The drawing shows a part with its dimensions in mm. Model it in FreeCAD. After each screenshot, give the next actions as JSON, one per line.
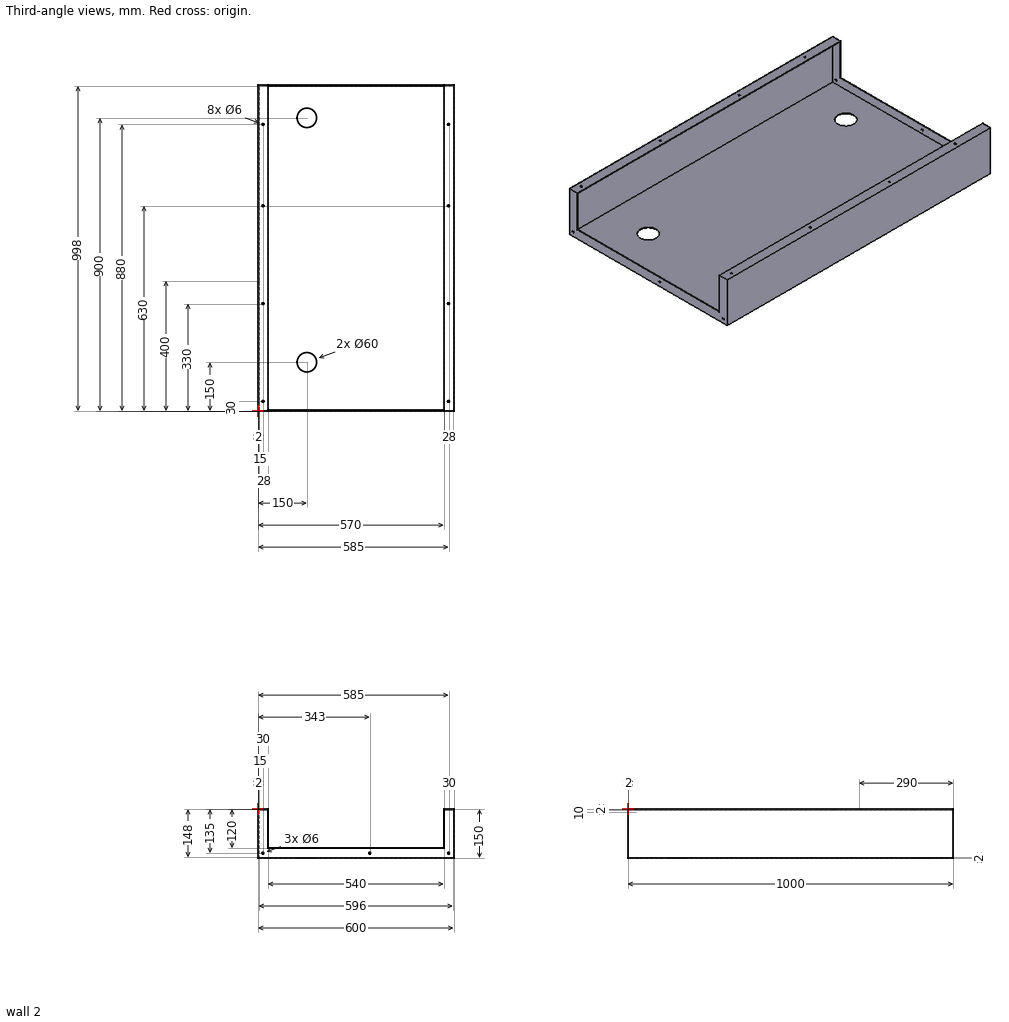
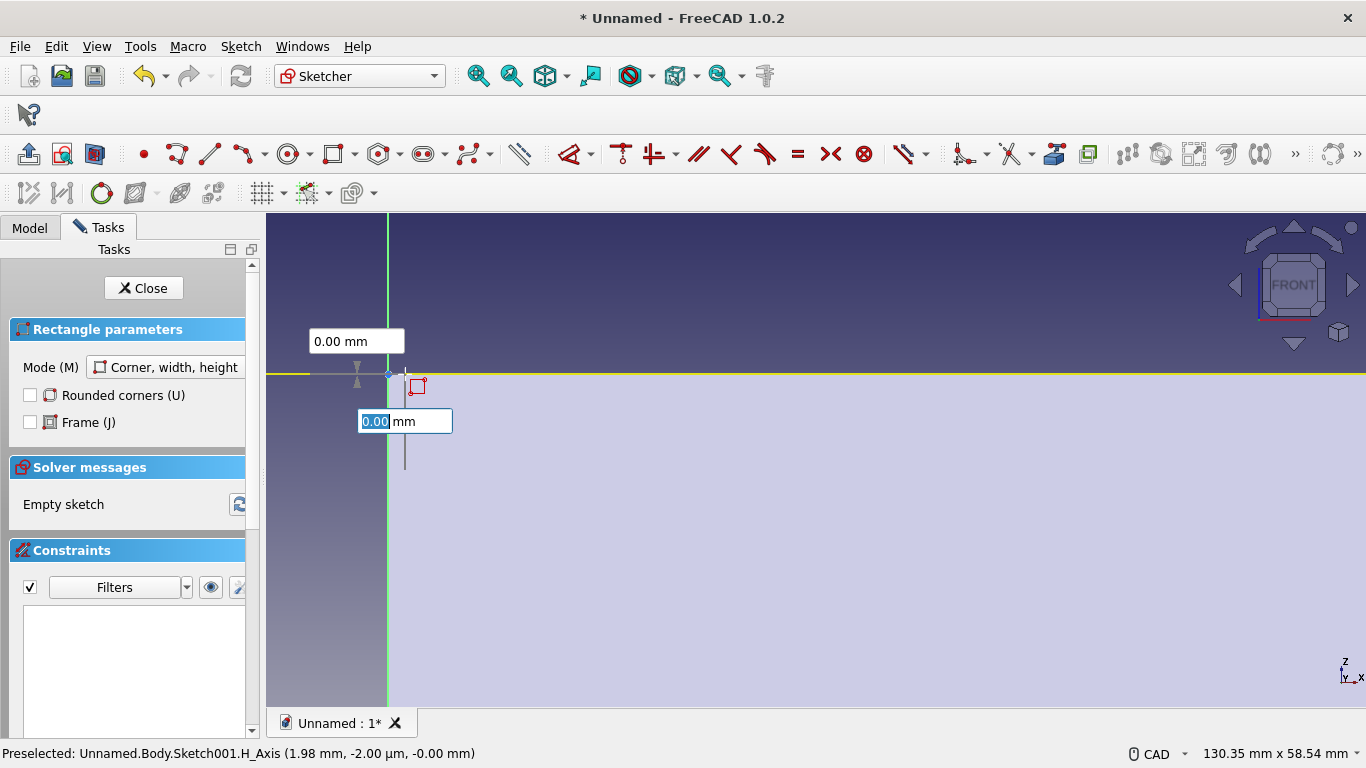
{"action": "scroll", "coordinate": [409, 376], "scroll_direction": "down", "scroll_amount": 10}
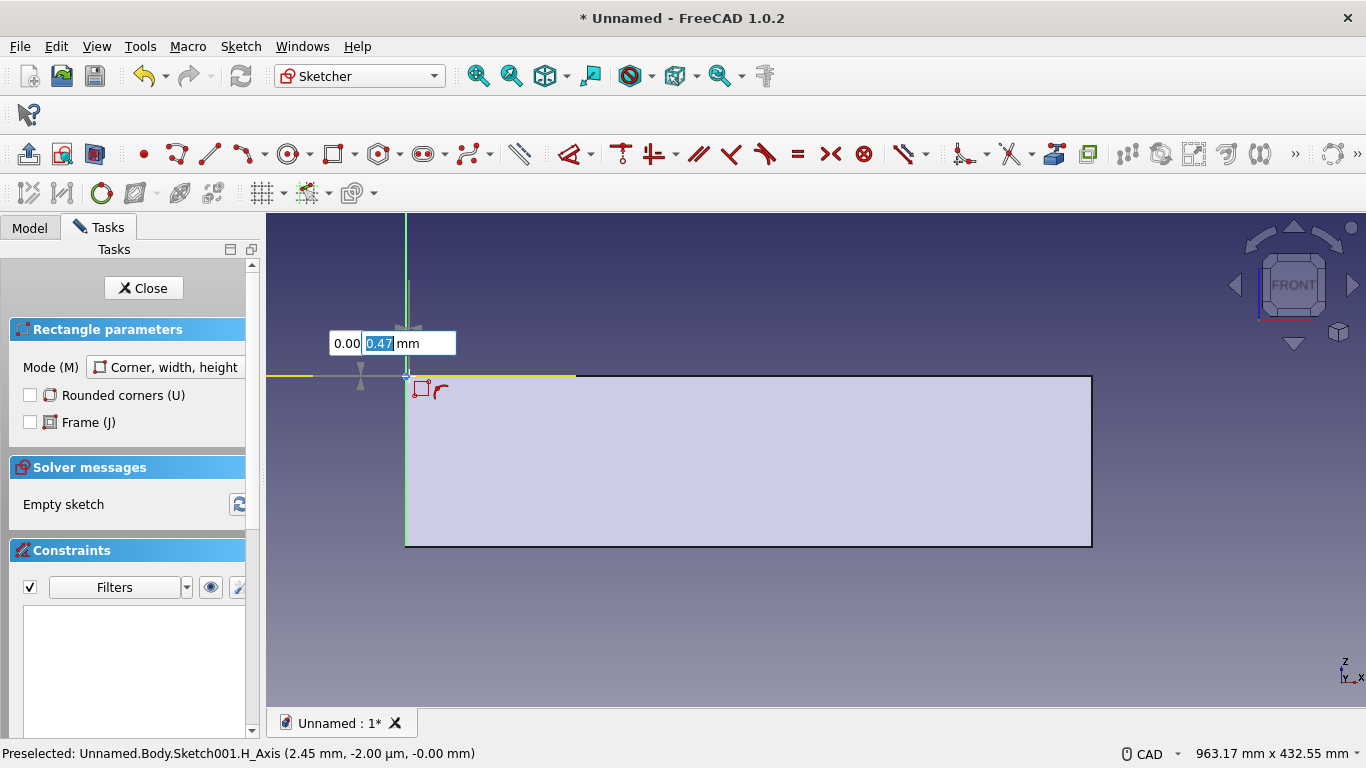
{"action": "left_click", "coordinate": [1089, 545]}
{"action": "key", "text": "Escape"}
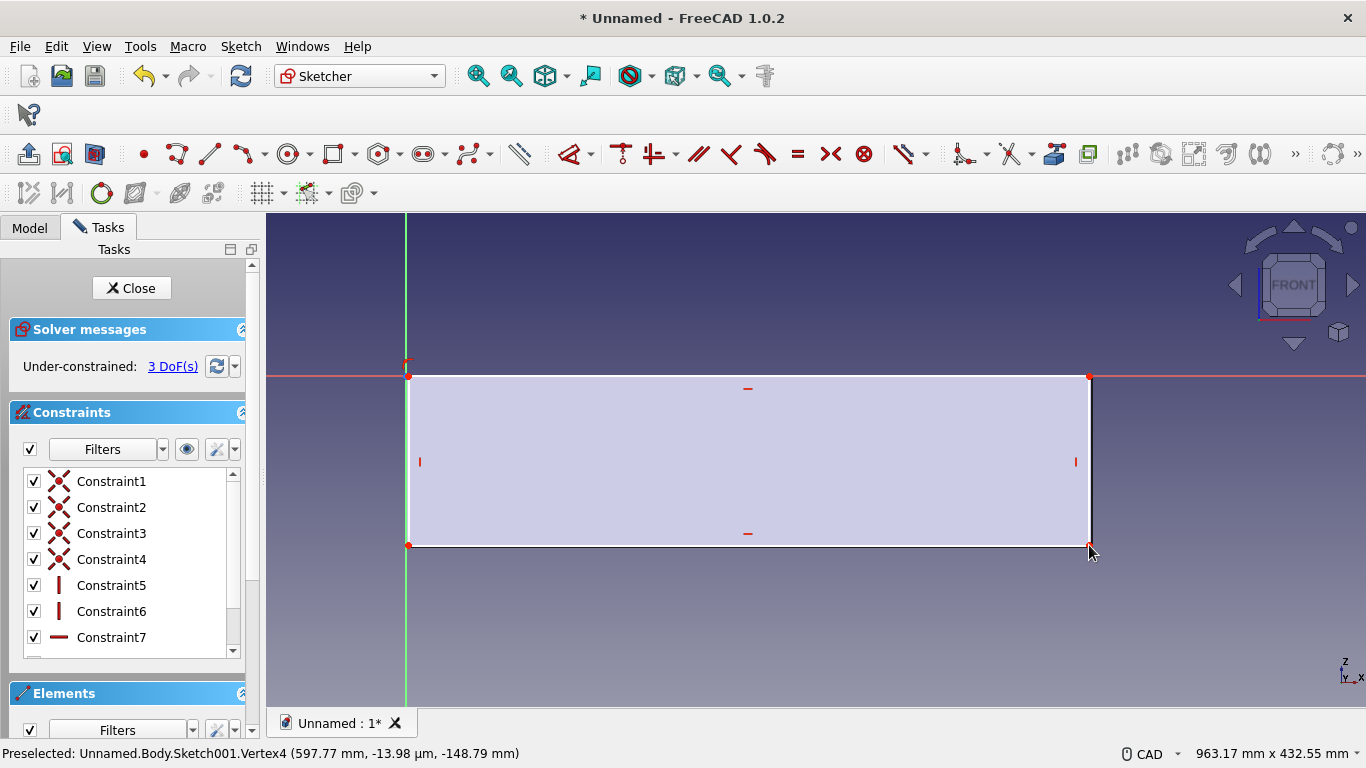
{"action": "scroll", "coordinate": [409, 376], "scroll_direction": "up", "scroll_amount": 15}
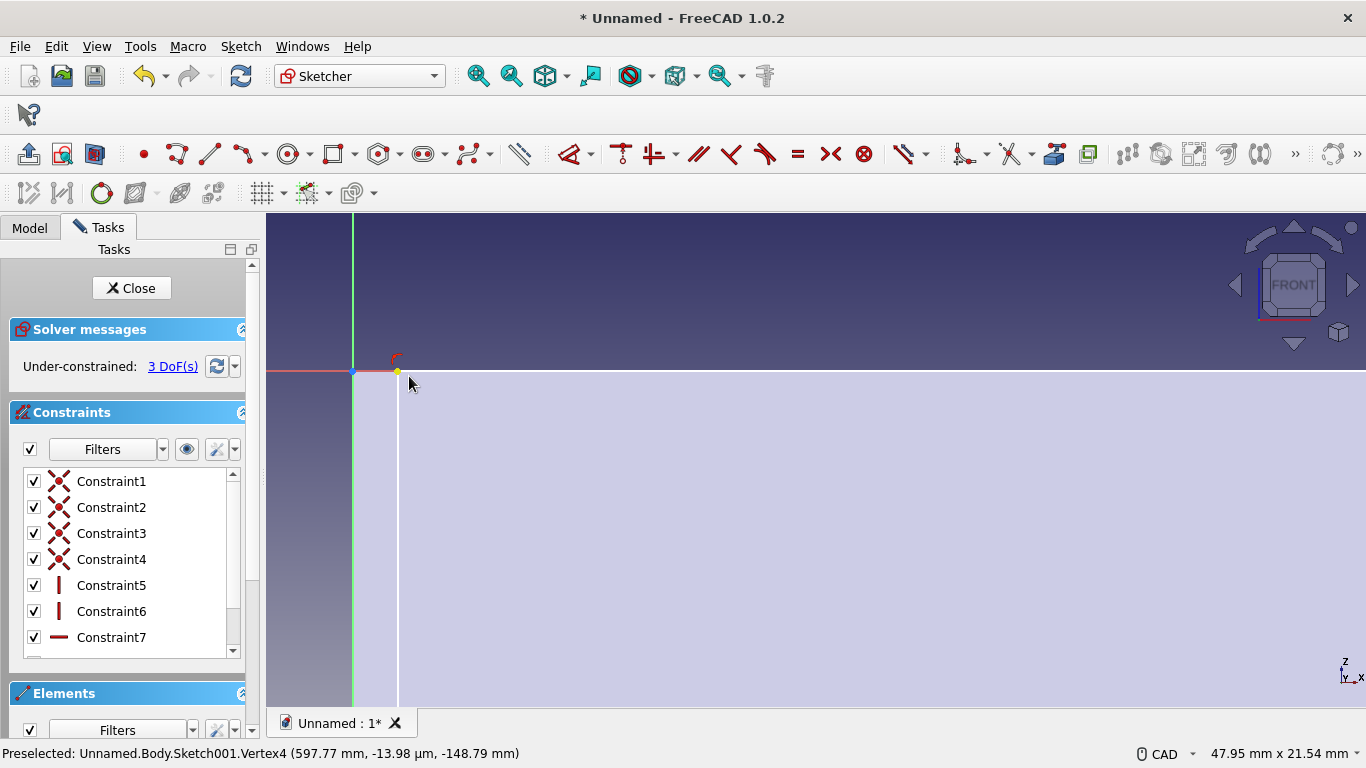
{"action": "left_click", "coordinate": [398, 371]}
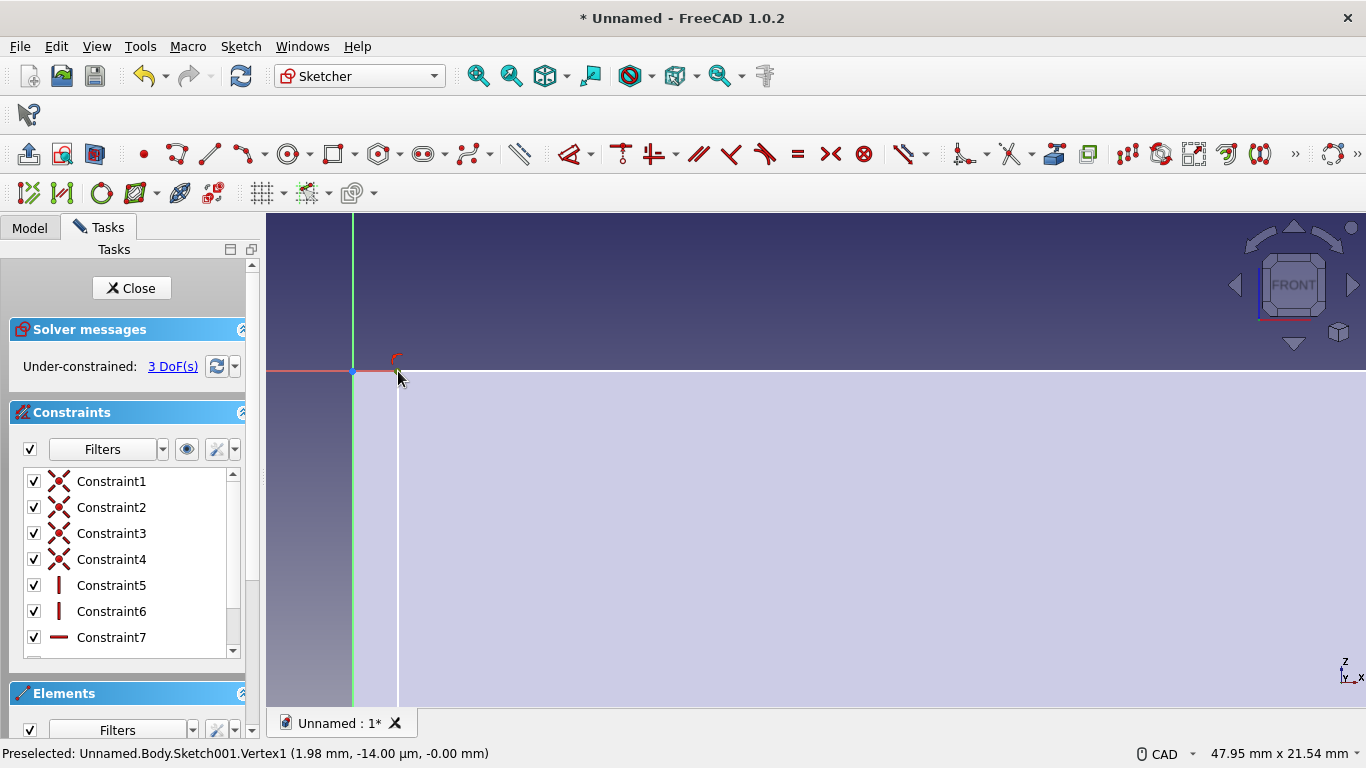
{"action": "left_click", "coordinate": [590, 154]}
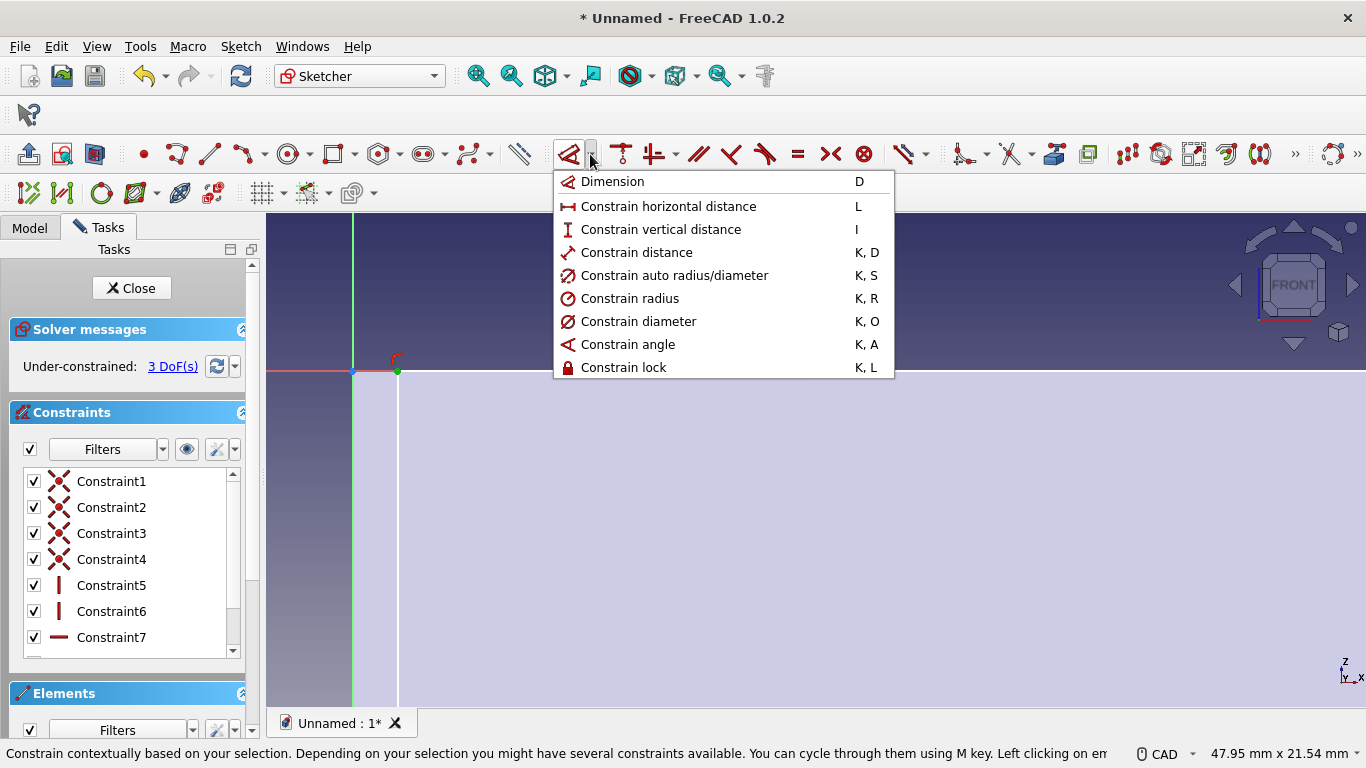
{"action": "left_click", "coordinate": [724, 206]}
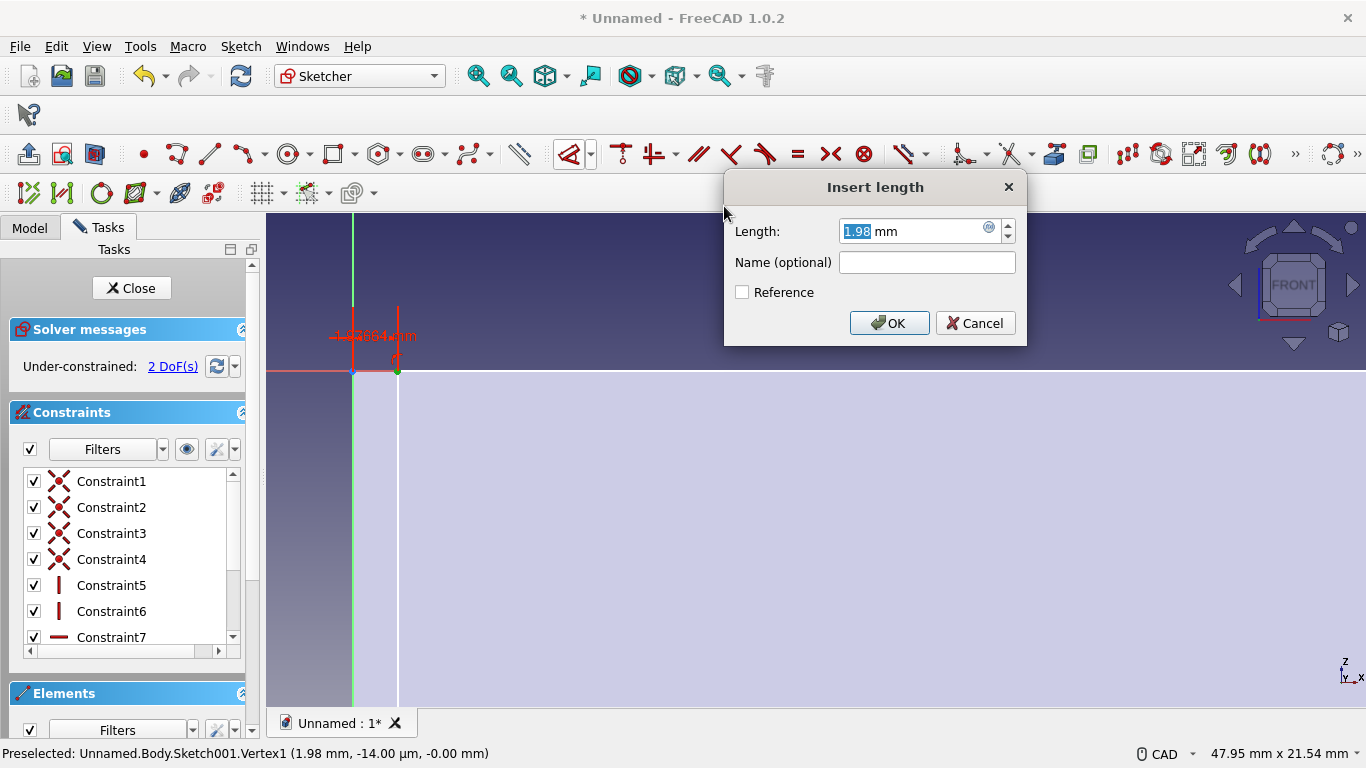
{"action": "type", "text": "2"}
{"action": "key", "text": "Return"}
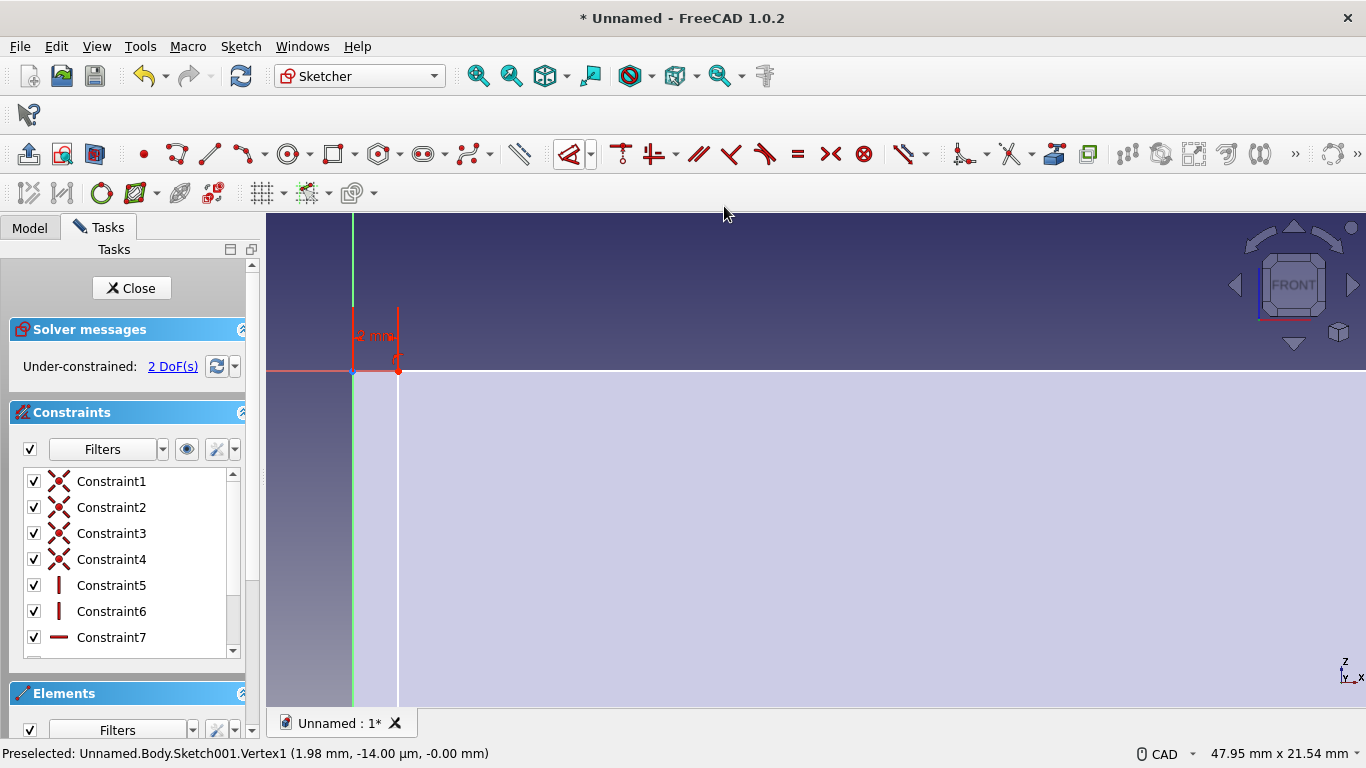
{"action": "scroll", "coordinate": [409, 376], "scroll_direction": "down", "scroll_amount": 15}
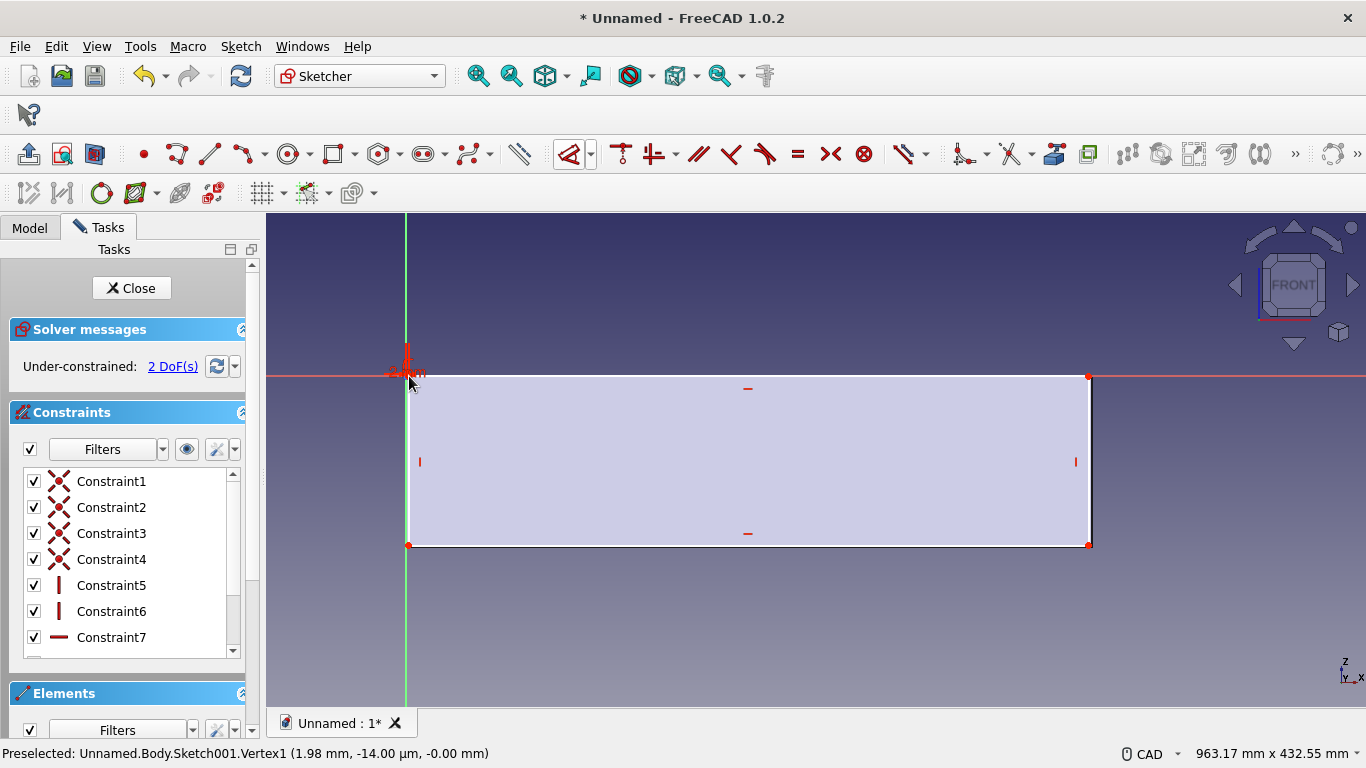
{"action": "scroll", "coordinate": [409, 427], "scroll_direction": "up", "scroll_amount": 9}